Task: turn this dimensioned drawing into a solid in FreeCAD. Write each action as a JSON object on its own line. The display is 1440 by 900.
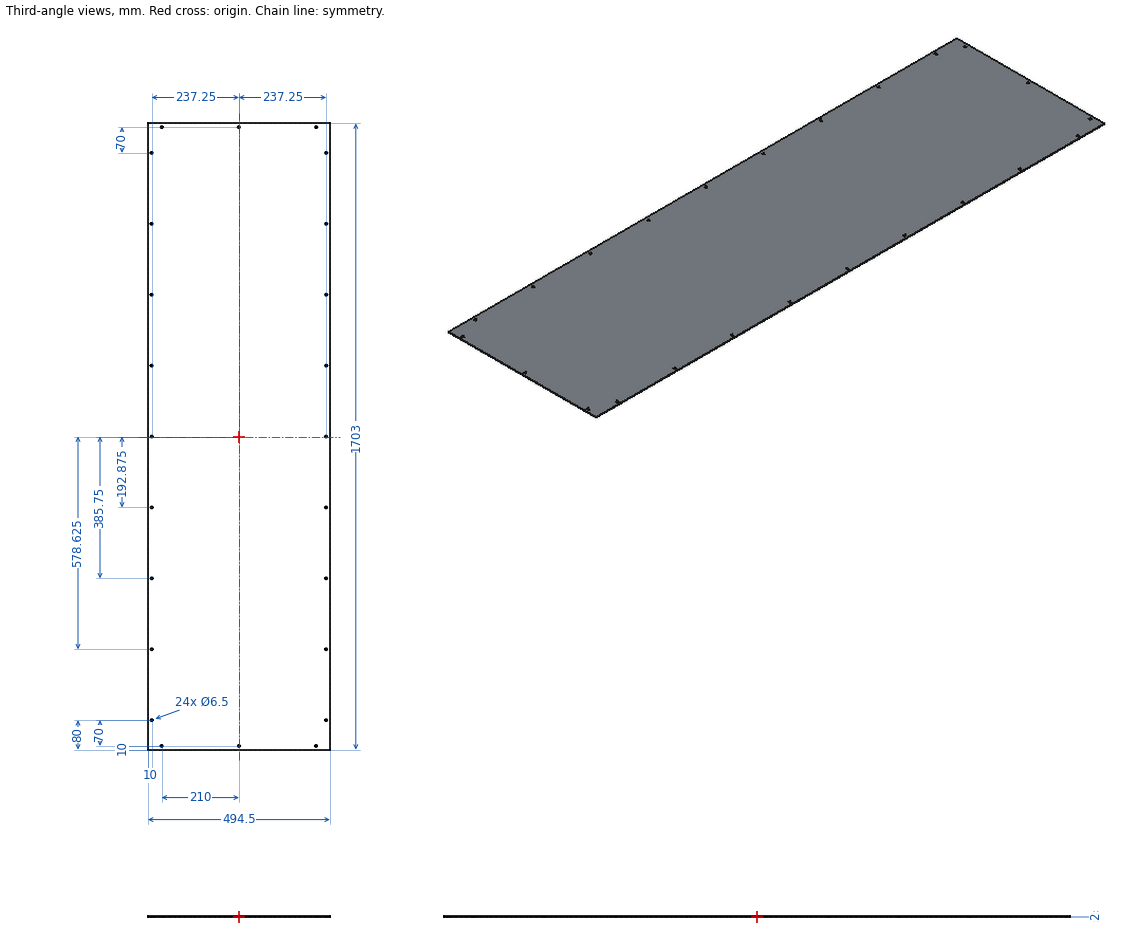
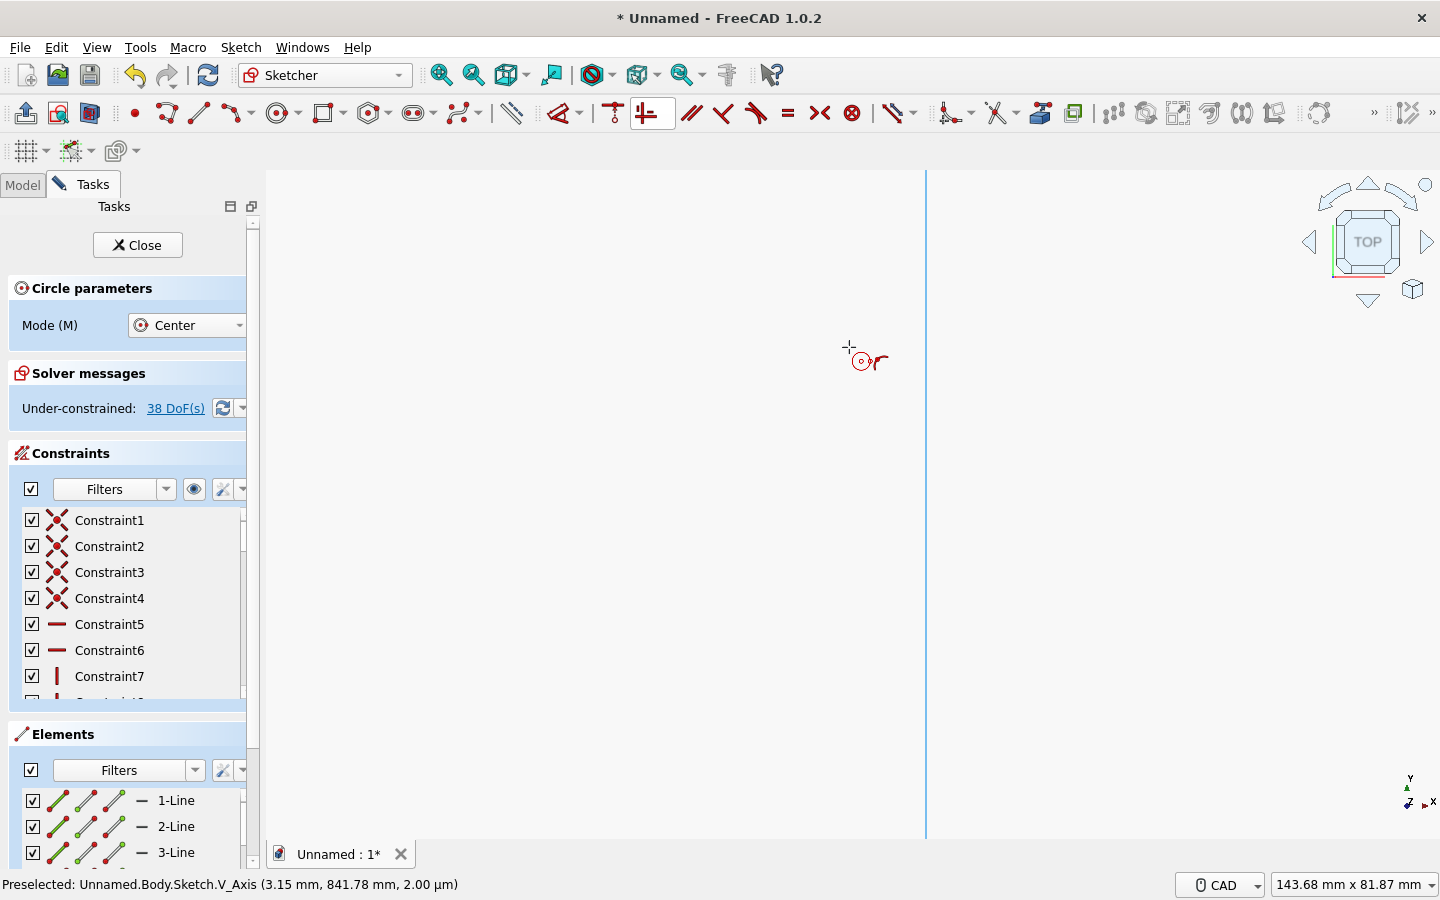
{"action": "scroll", "coordinate": [849, 347], "scroll_direction": "down", "scroll_amount": 17}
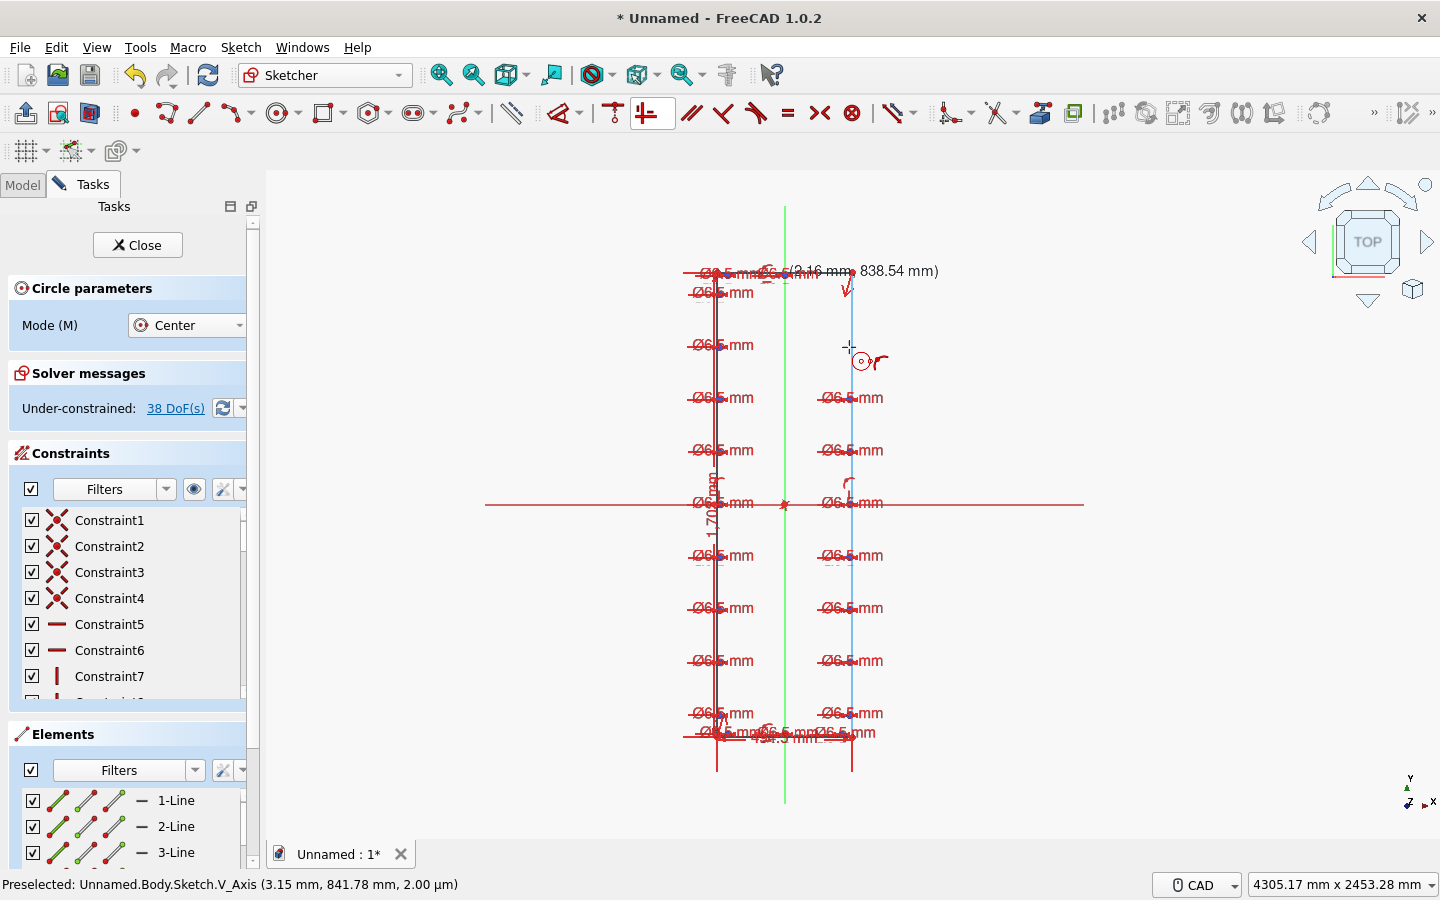
{"action": "scroll", "coordinate": [849, 347], "scroll_direction": "up", "scroll_amount": 9}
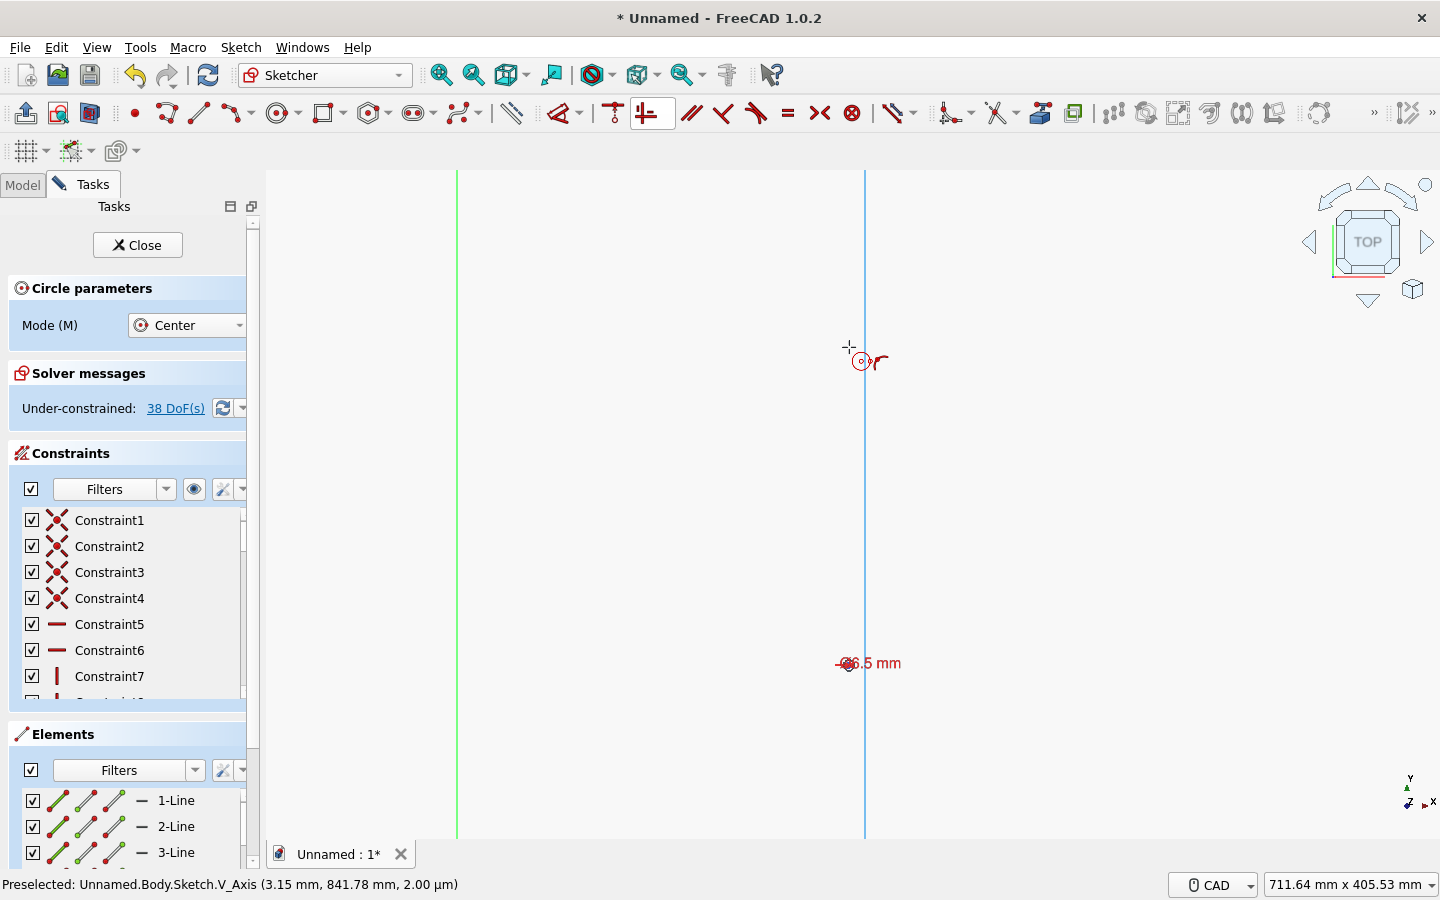
{"action": "left_click", "coordinate": [849, 346]}
{"action": "mouse_move", "coordinate": [845, 342]}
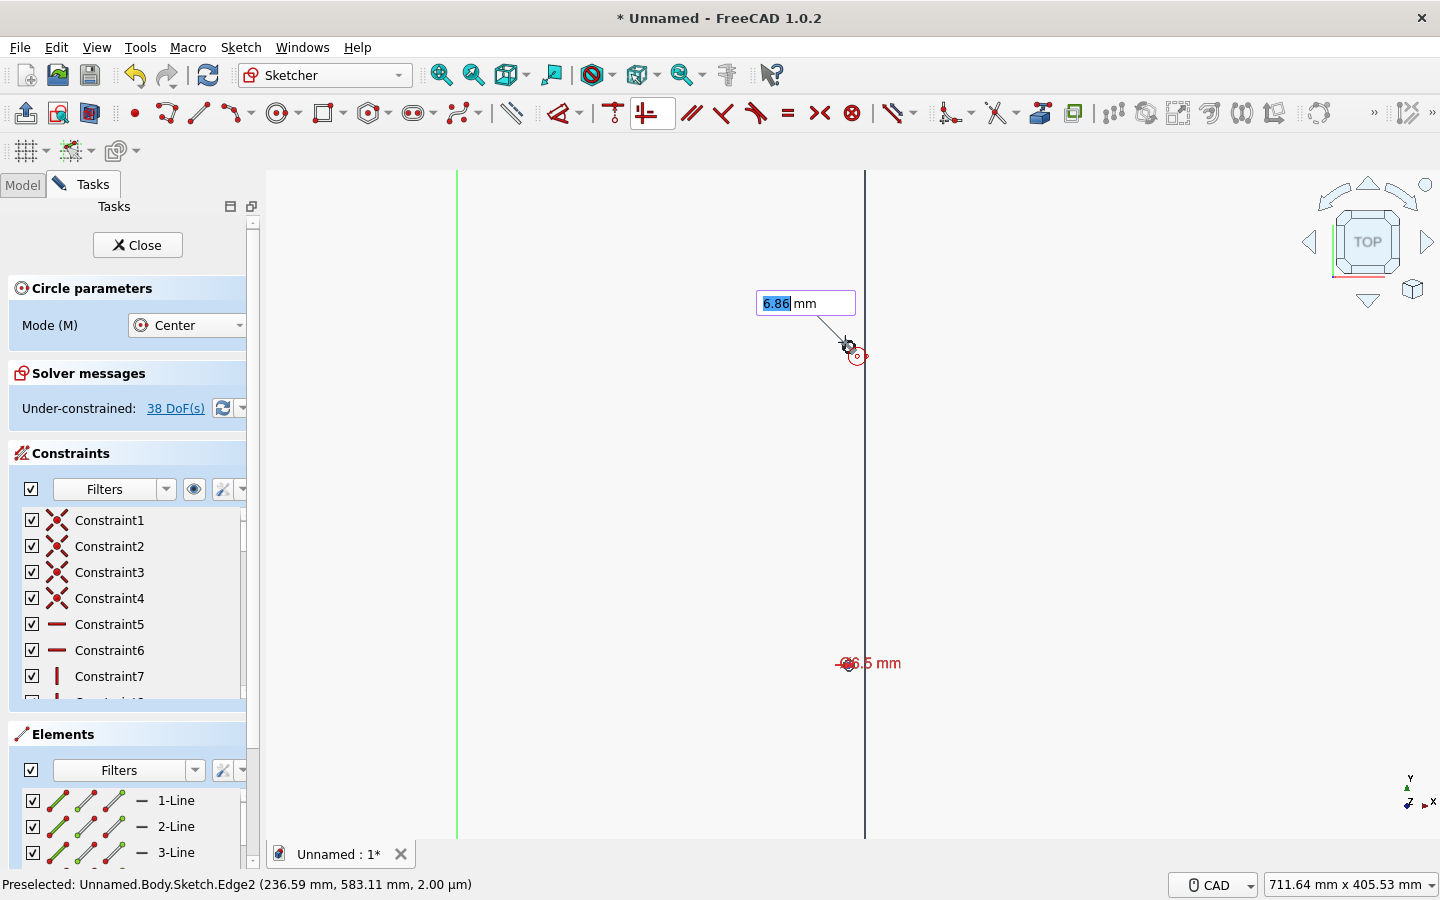
{"action": "type", "text": "6.5"}
{"action": "key", "text": "Return"}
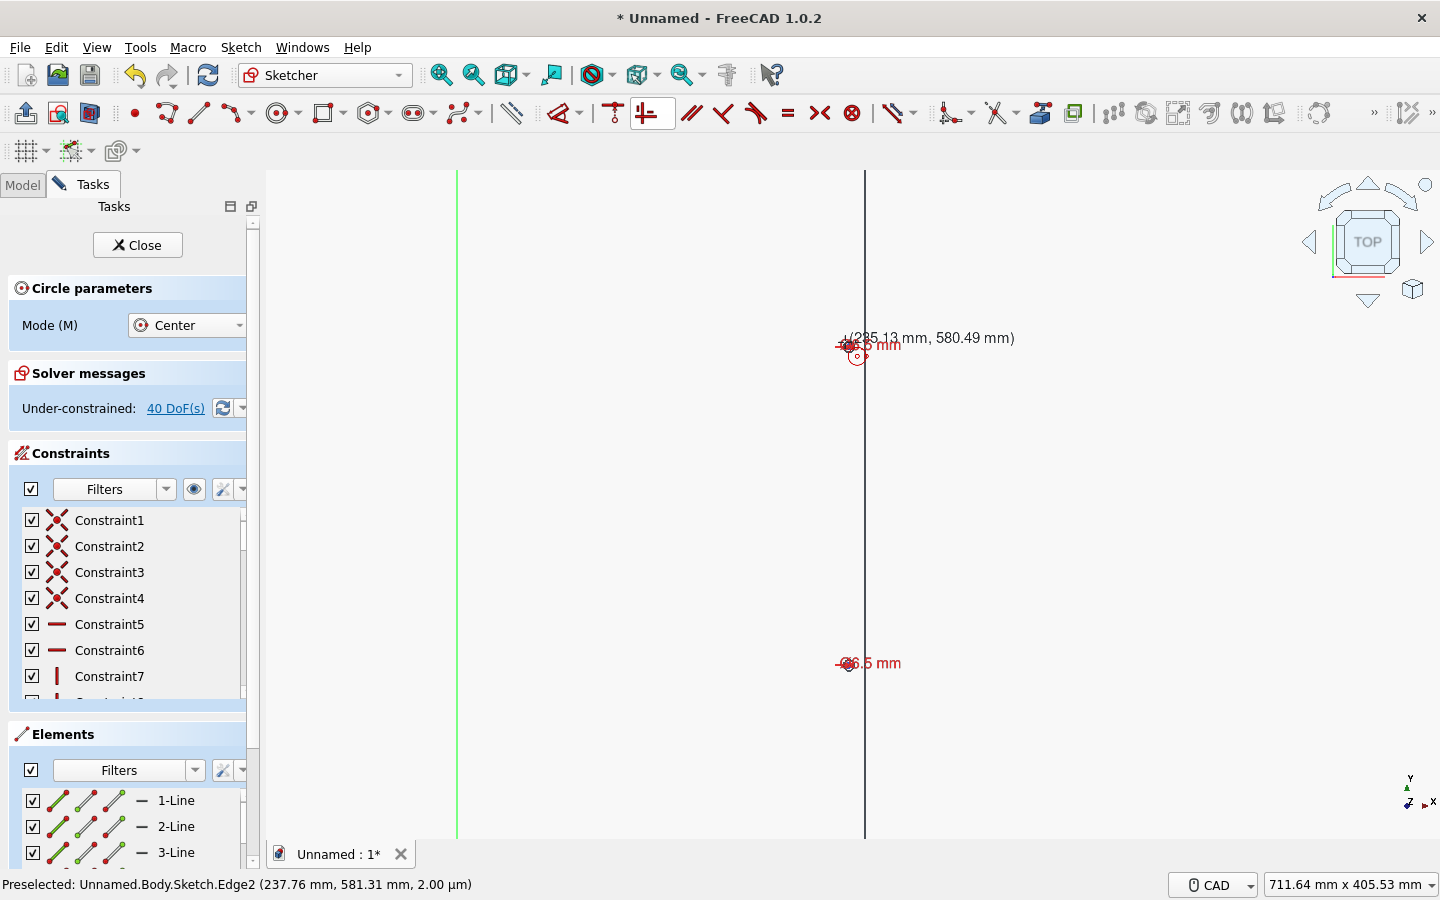
{"action": "scroll", "coordinate": [849, 347], "scroll_direction": "down", "scroll_amount": 9}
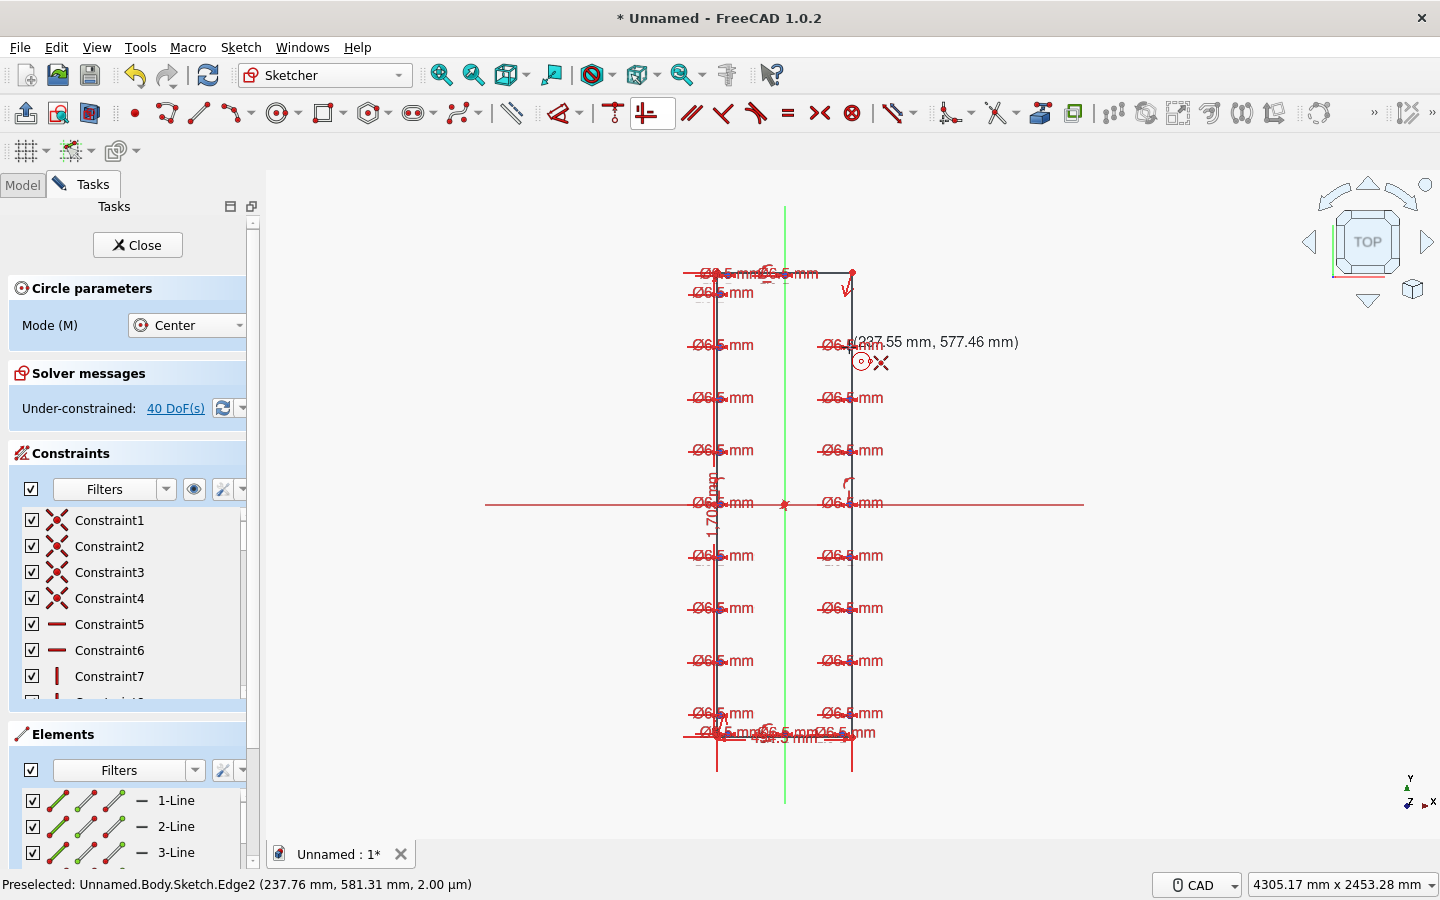
{"action": "scroll", "coordinate": [842, 275], "scroll_direction": "up", "scroll_amount": 17}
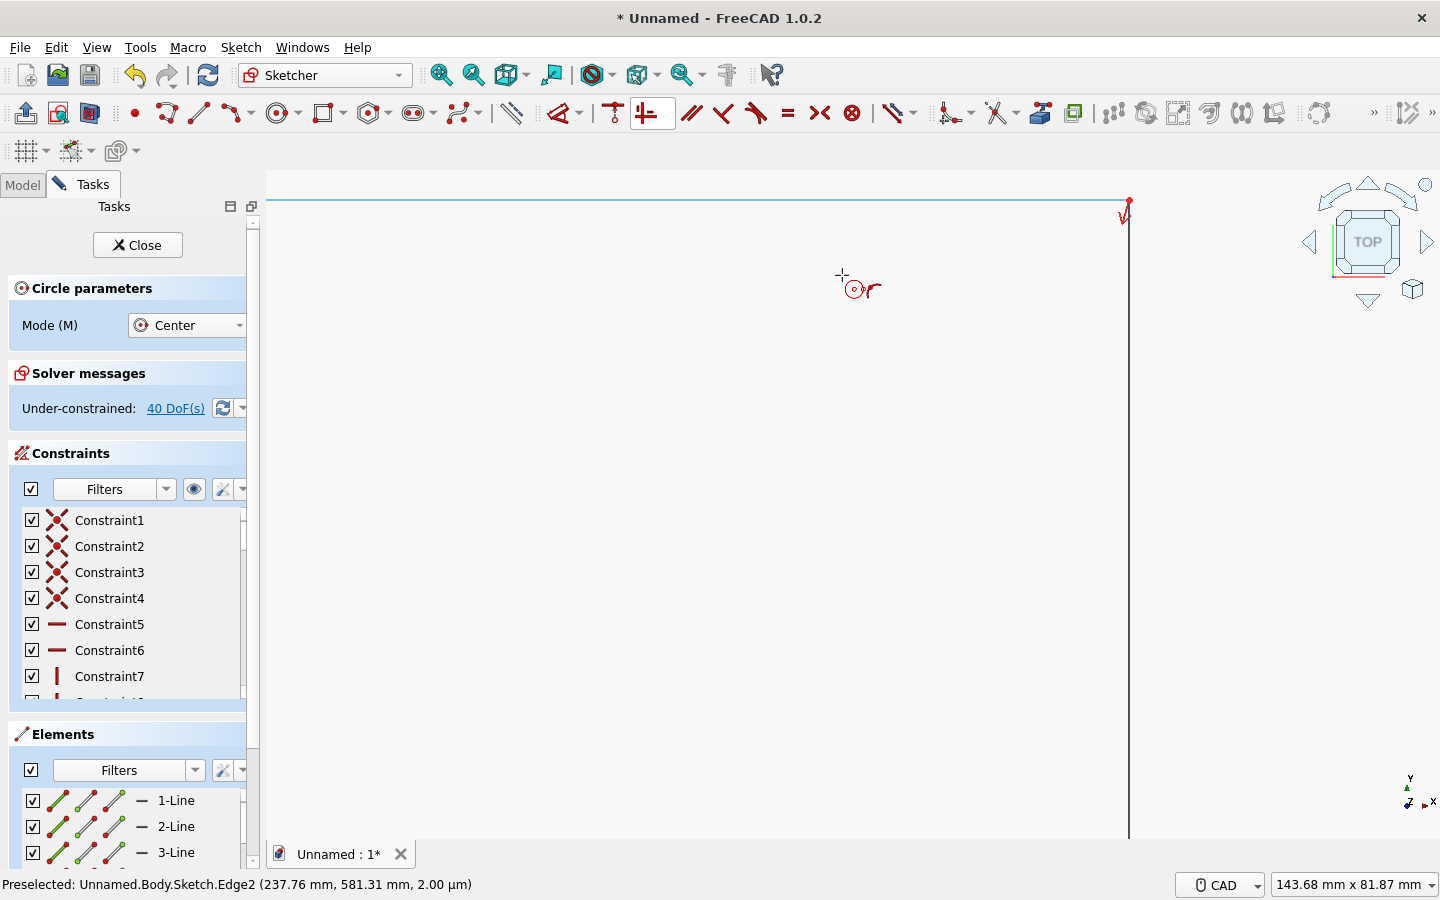
{"action": "scroll", "coordinate": [842, 275], "scroll_direction": "down", "scroll_amount": 17}